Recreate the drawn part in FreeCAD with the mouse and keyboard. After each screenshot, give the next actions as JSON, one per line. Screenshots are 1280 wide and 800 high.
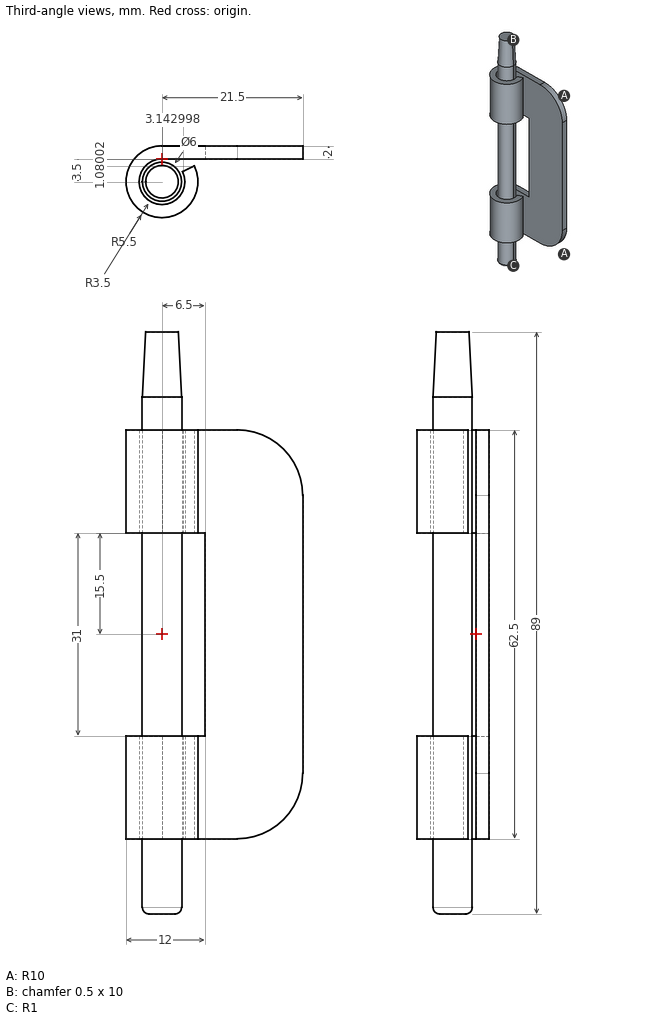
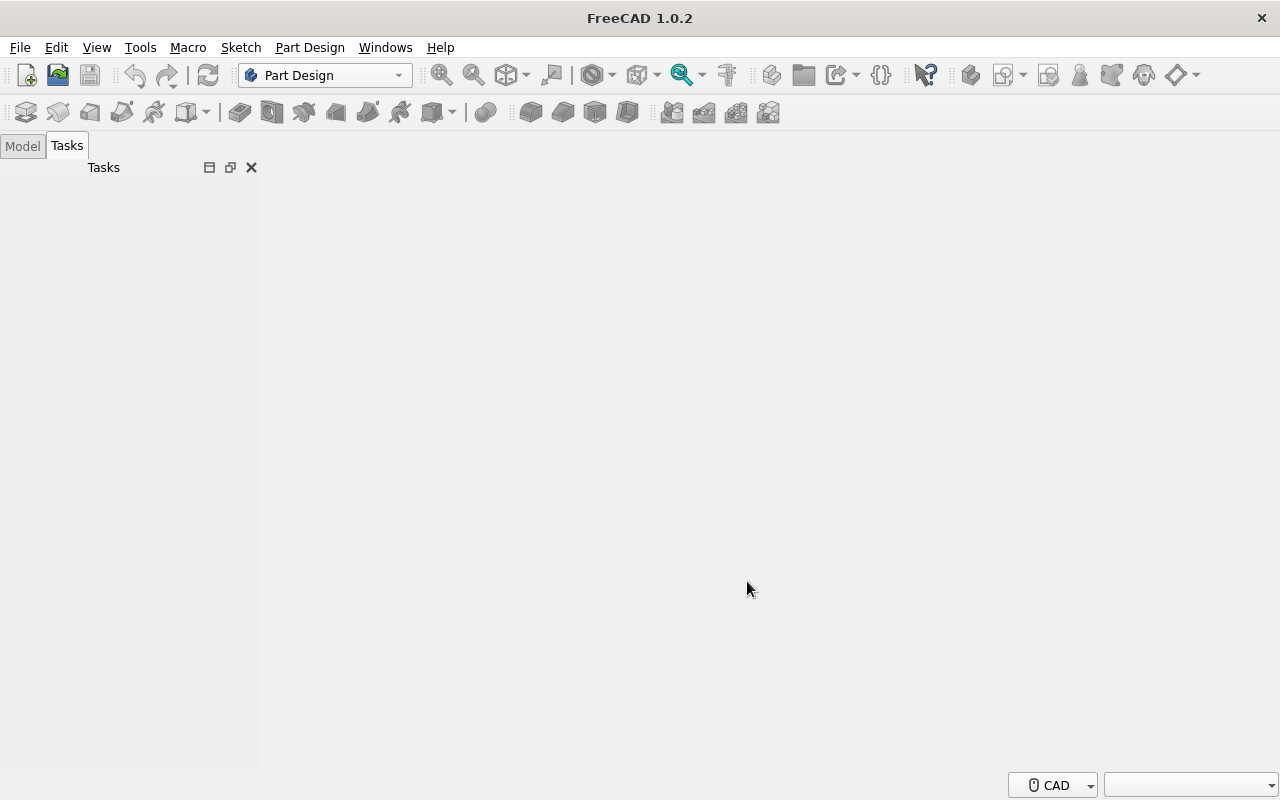
{"action": "key", "text": "ctrl+n"}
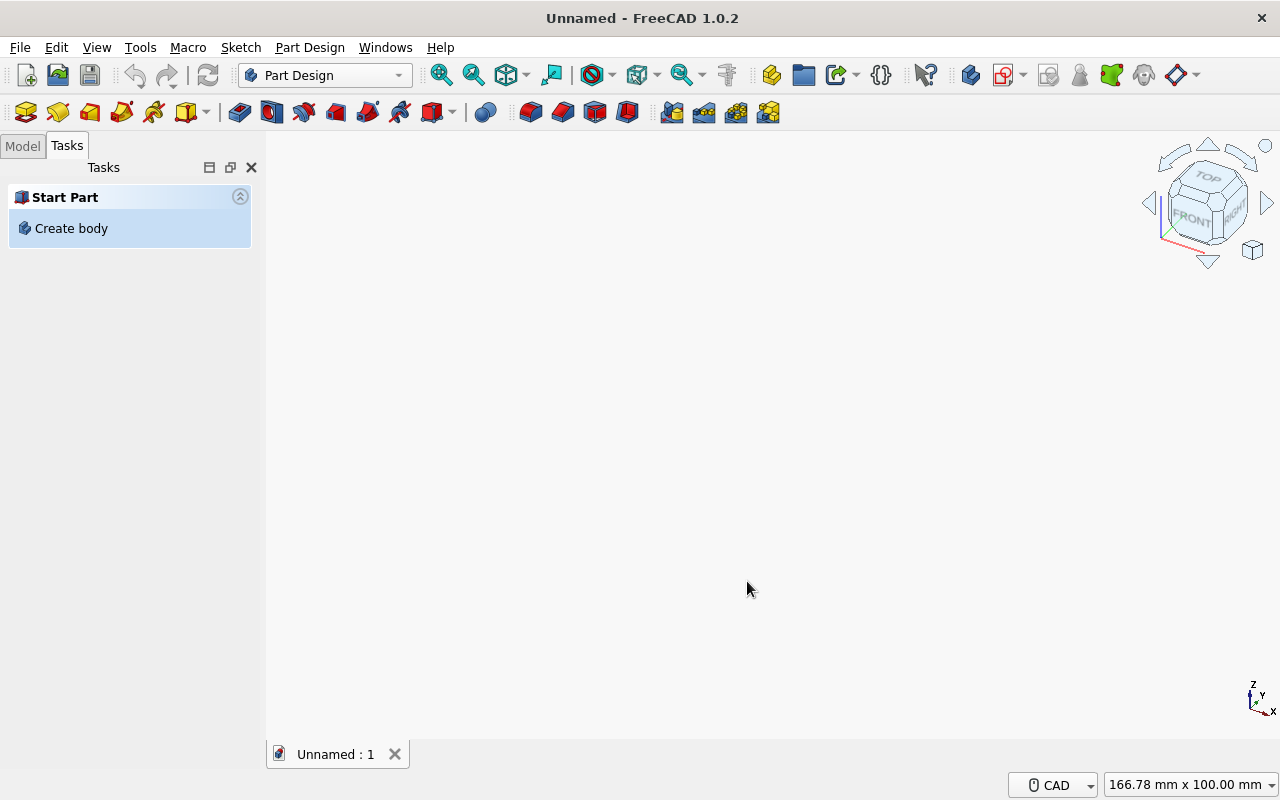
{"action": "left_click", "coordinate": [1004, 76]}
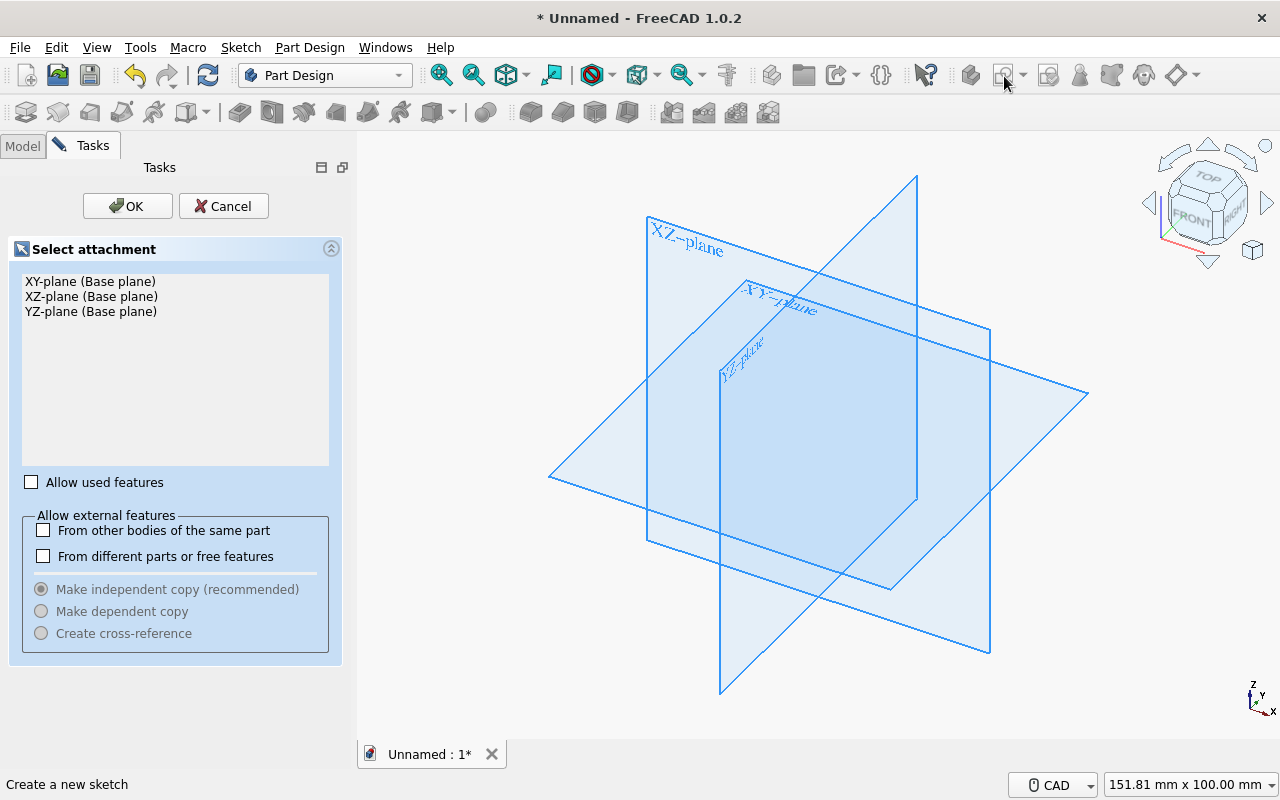
{"action": "left_click", "coordinate": [82, 282]}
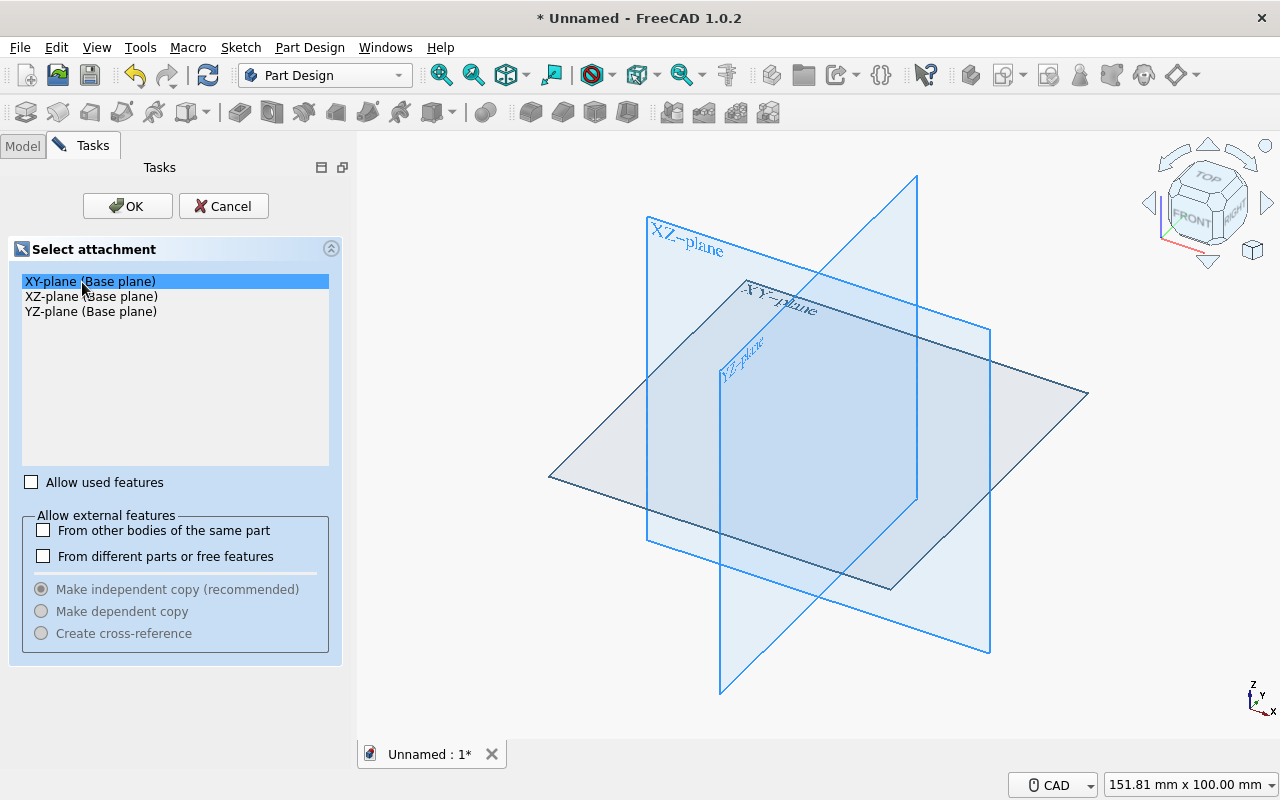
{"action": "left_click", "coordinate": [128, 206]}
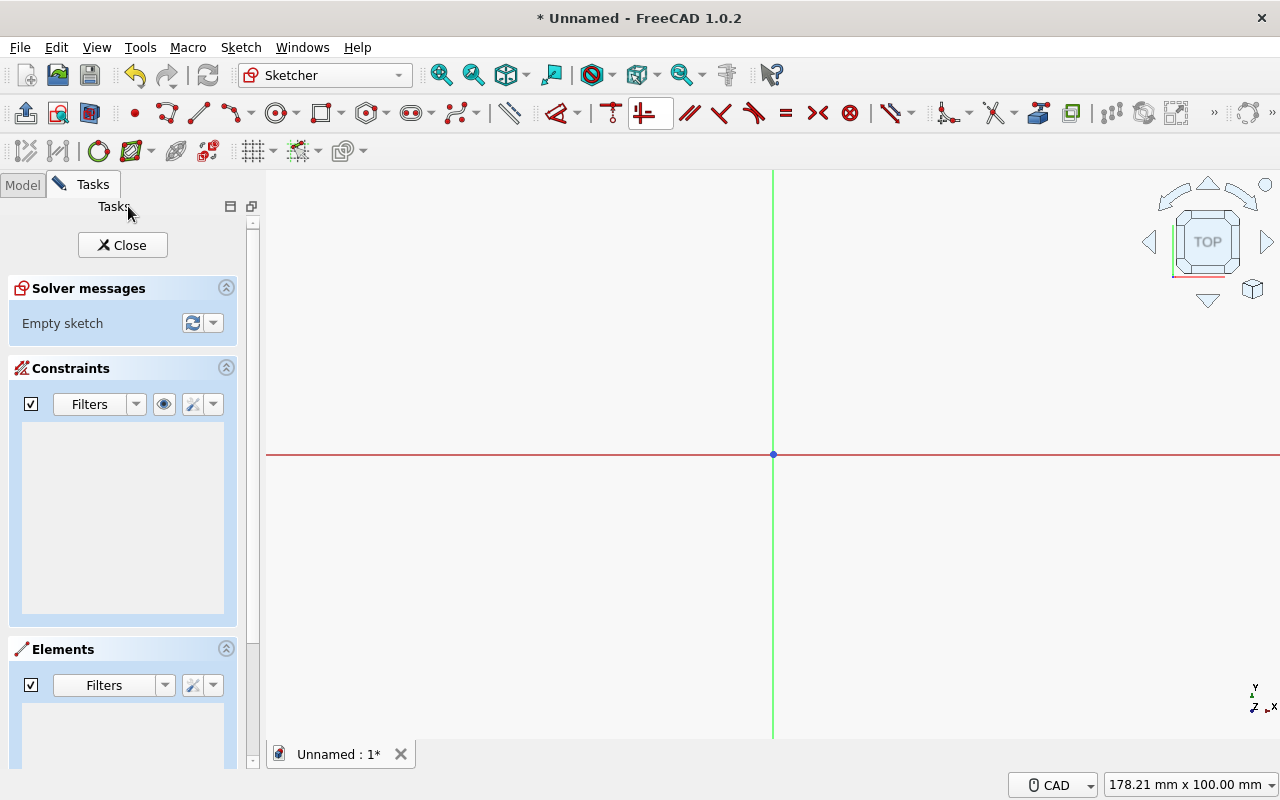
{"action": "scroll", "coordinate": [866, 478], "scroll_direction": "up", "scroll_amount": 7}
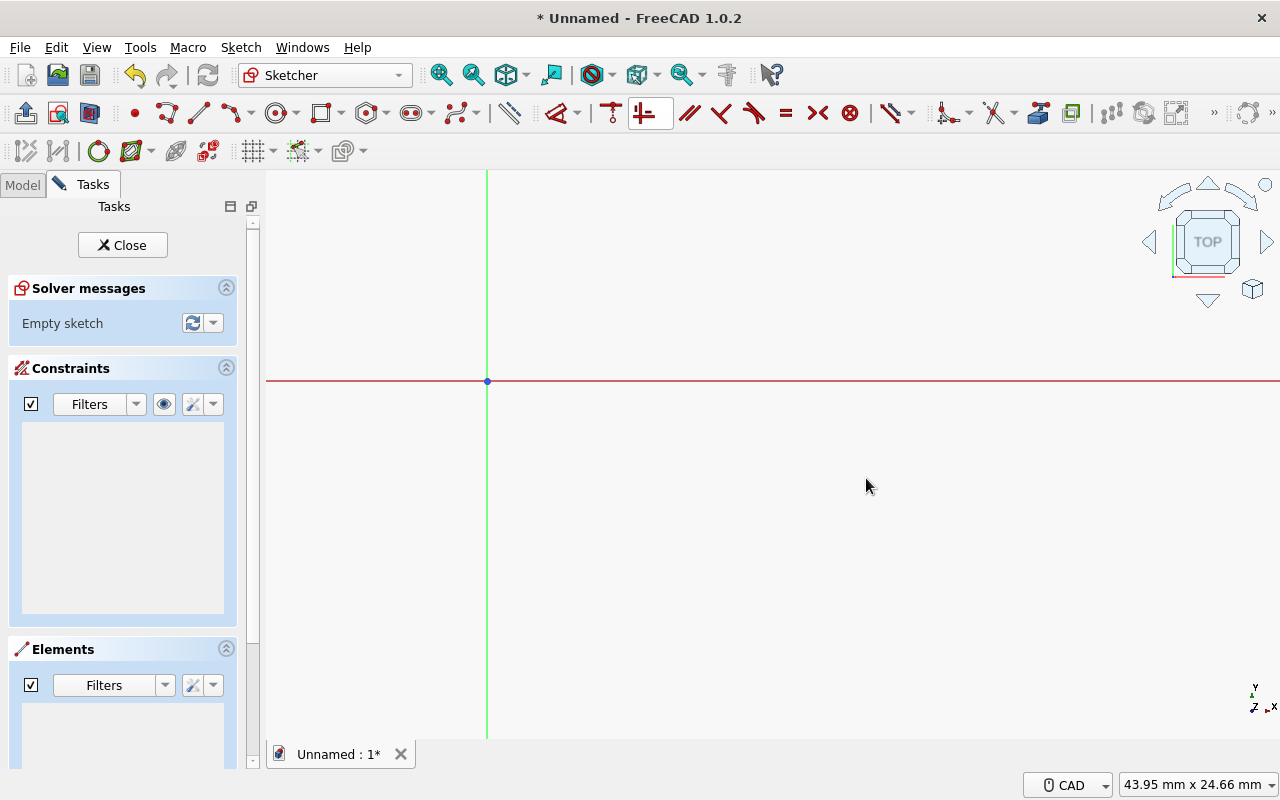
{"action": "key", "text": "g m"}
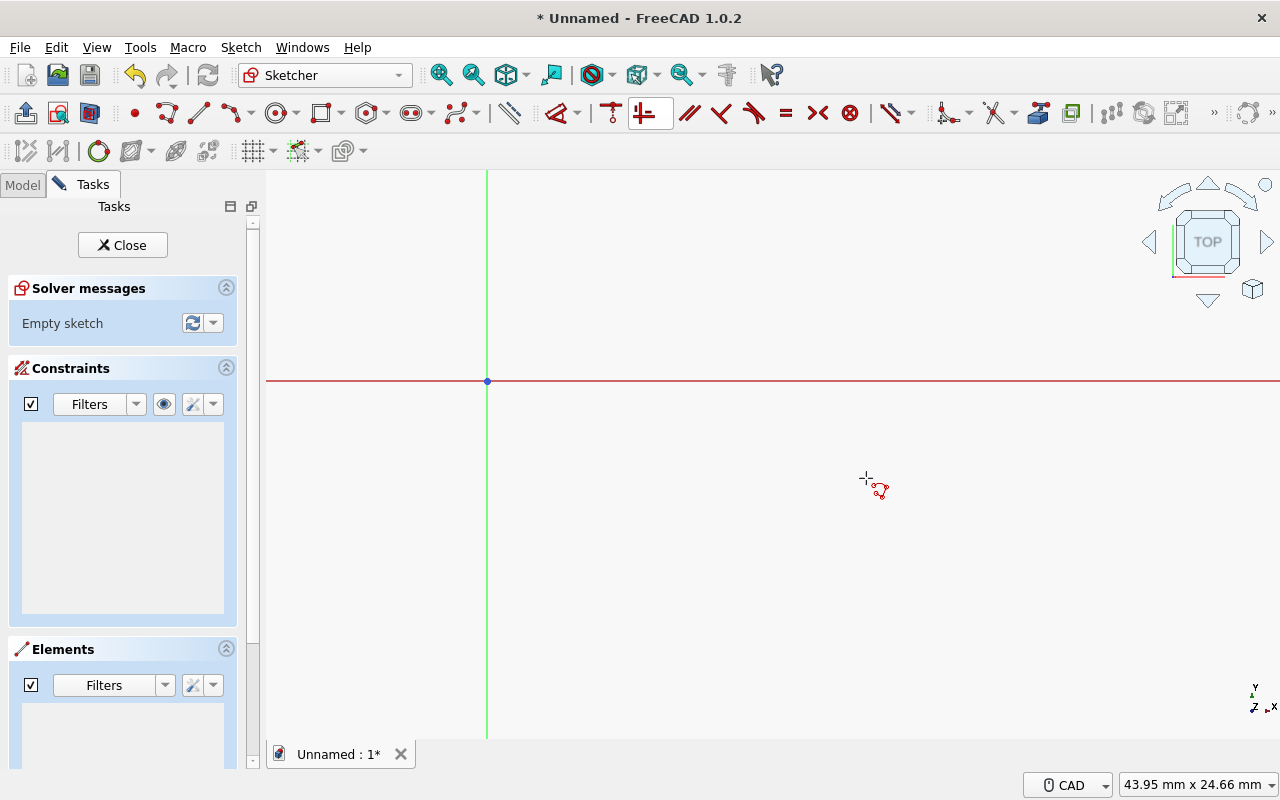
{"action": "left_click", "coordinate": [487, 381]}
{"action": "left_click", "coordinate": [983, 390]}
{"action": "left_click", "coordinate": [983, 335]}
{"action": "left_click", "coordinate": [487, 335]}
{"action": "right_click", "coordinate": [487, 335]}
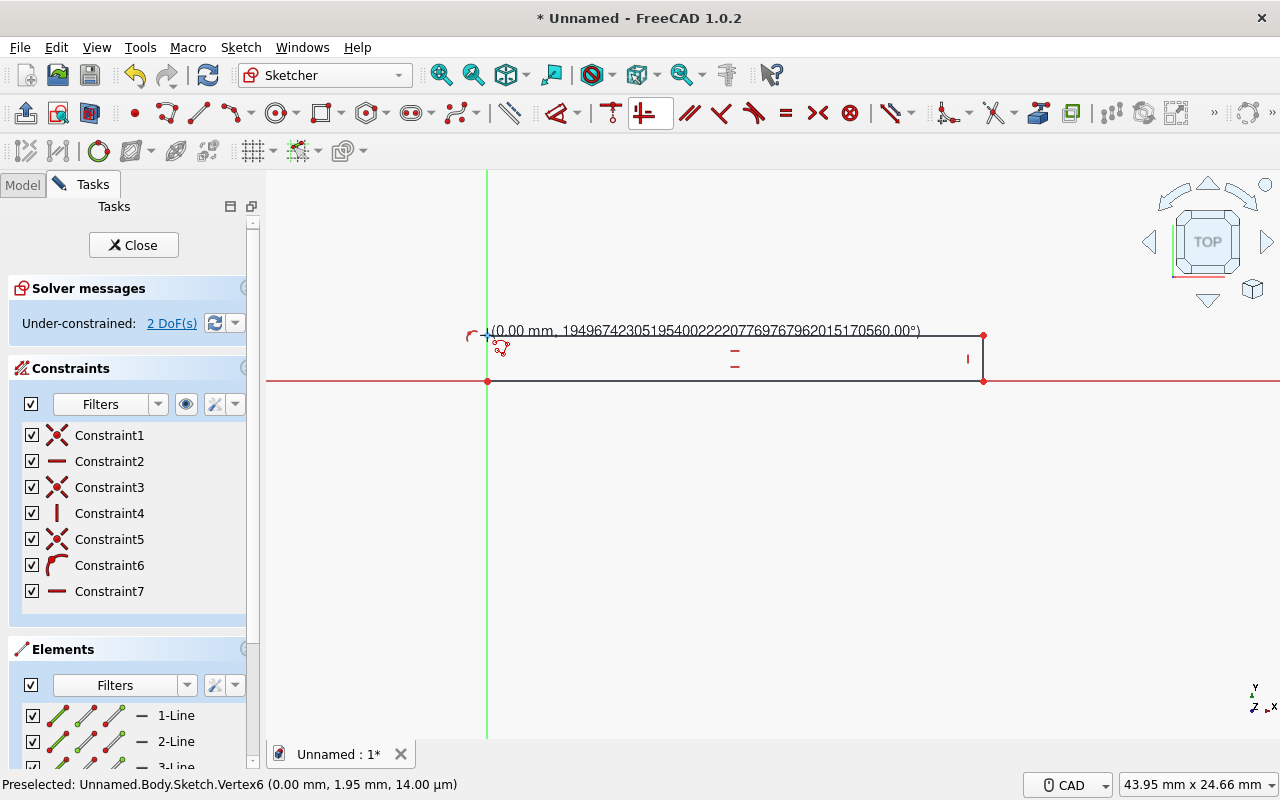
{"action": "key", "text": "g l"}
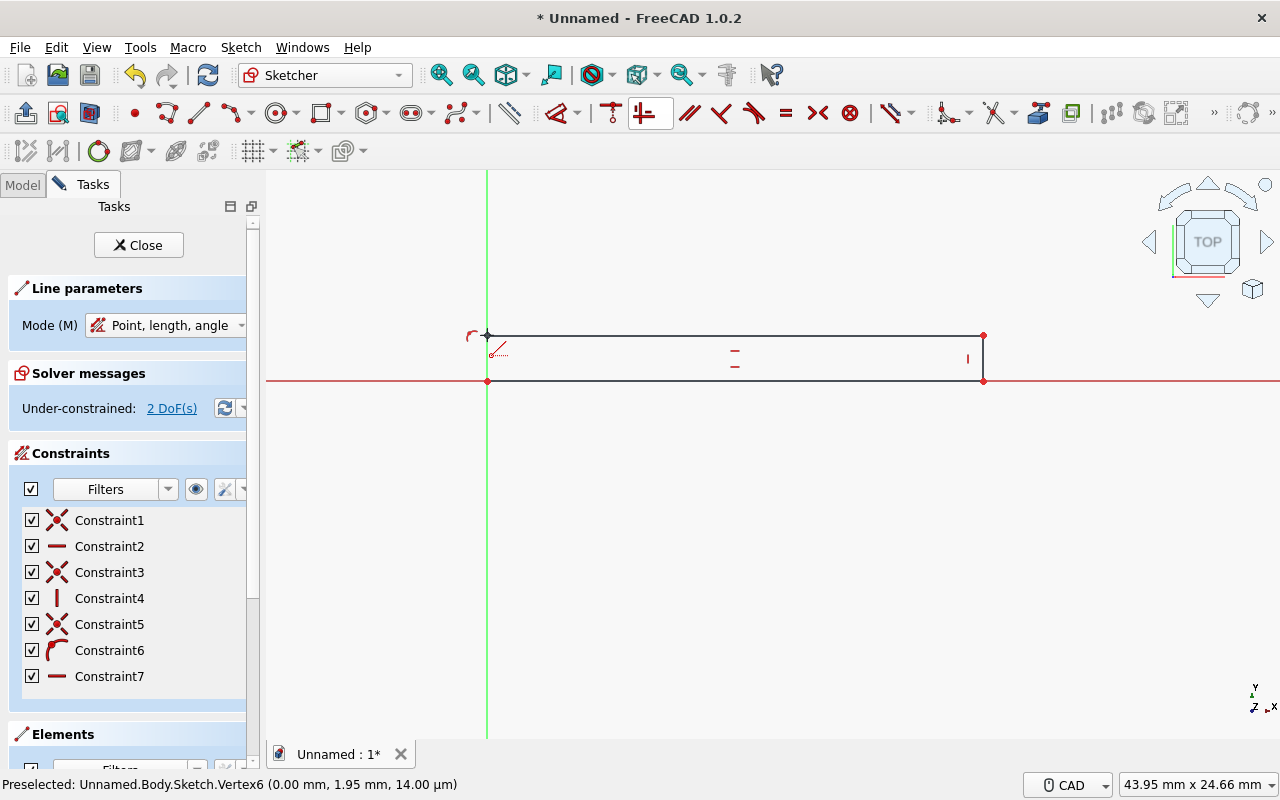
{"action": "left_click", "coordinate": [601, 406]}
{"action": "left_click", "coordinate": [560, 426]}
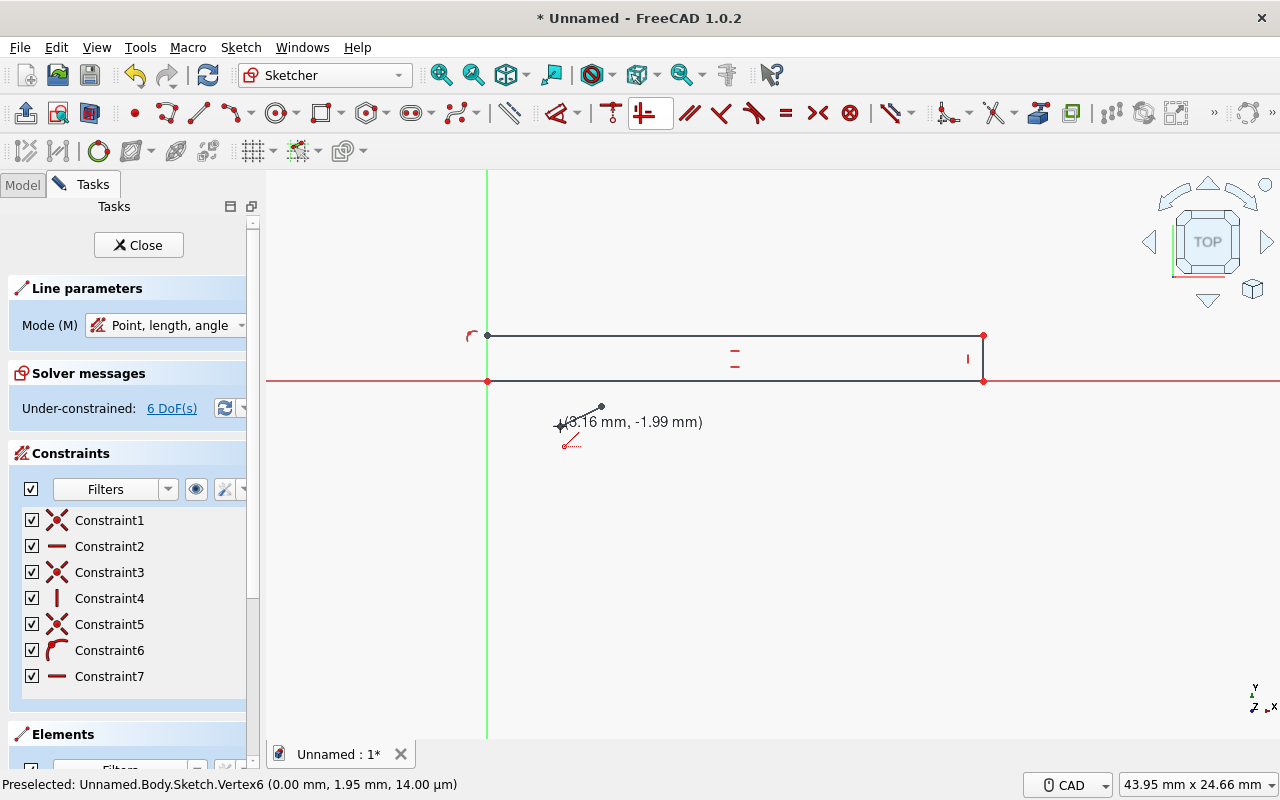
{"action": "key", "text": "g 3 a"}